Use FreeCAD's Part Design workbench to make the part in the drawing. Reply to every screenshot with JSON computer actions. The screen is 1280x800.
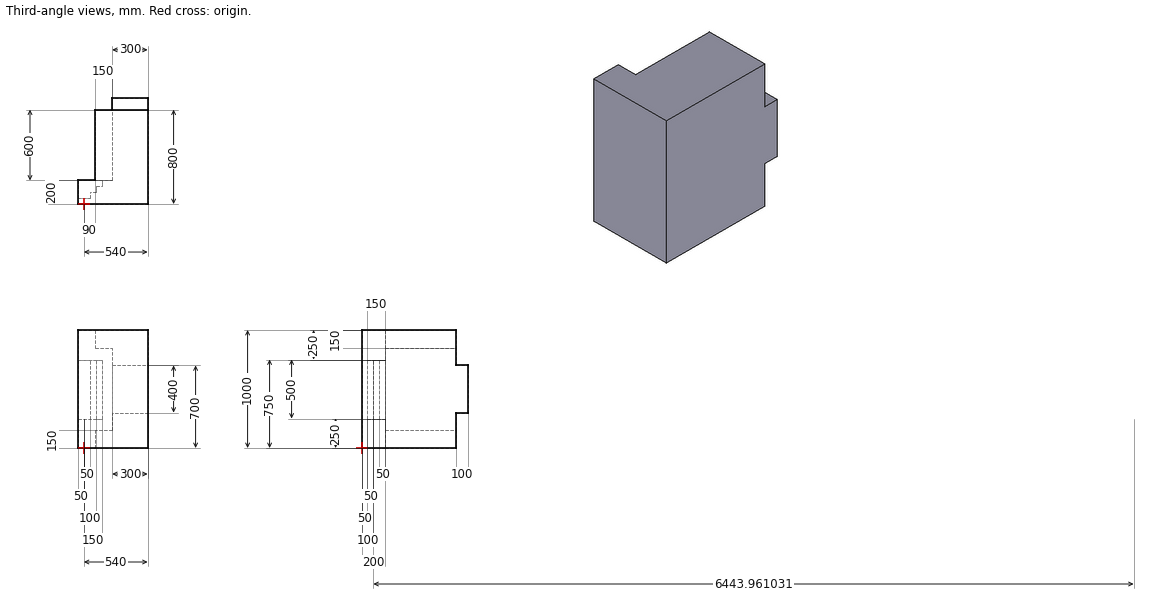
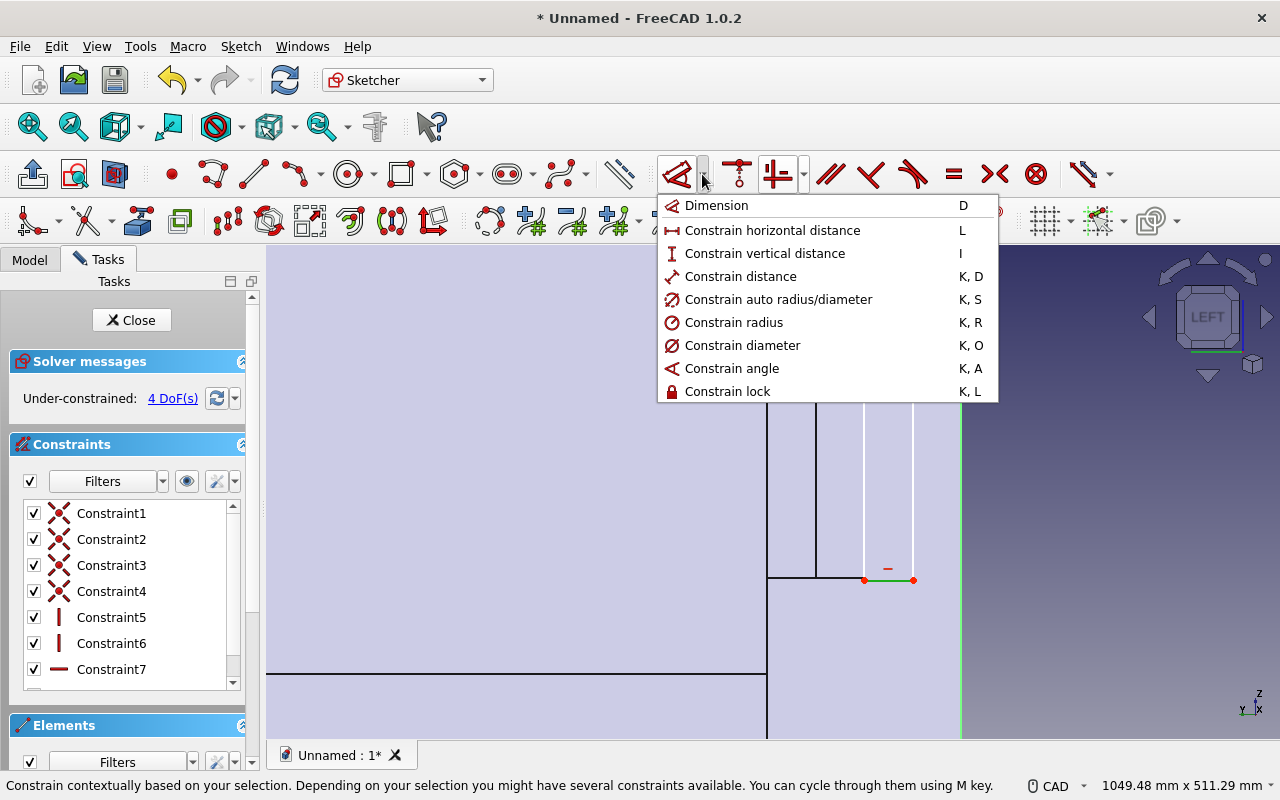
{"action": "left_click", "coordinate": [828, 230]}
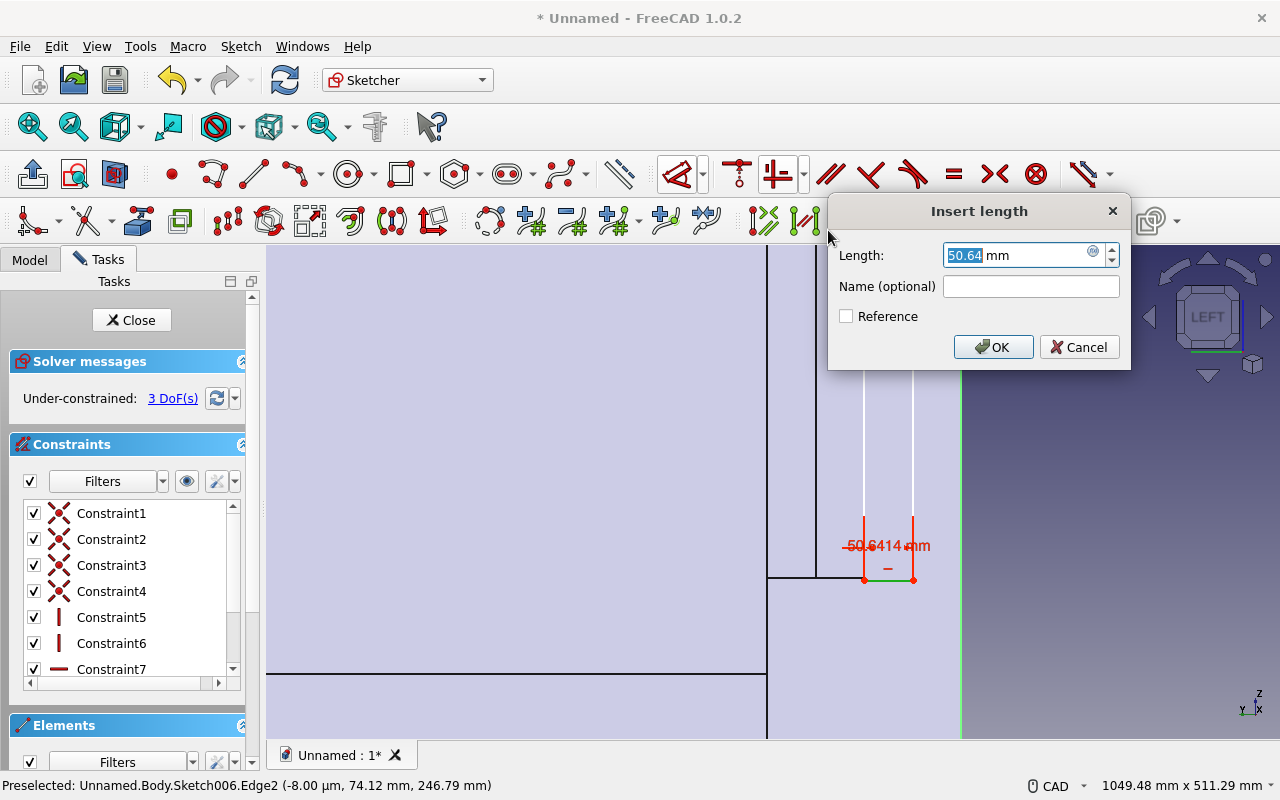
{"action": "type", "text": "50"}
{"action": "key", "text": "Return"}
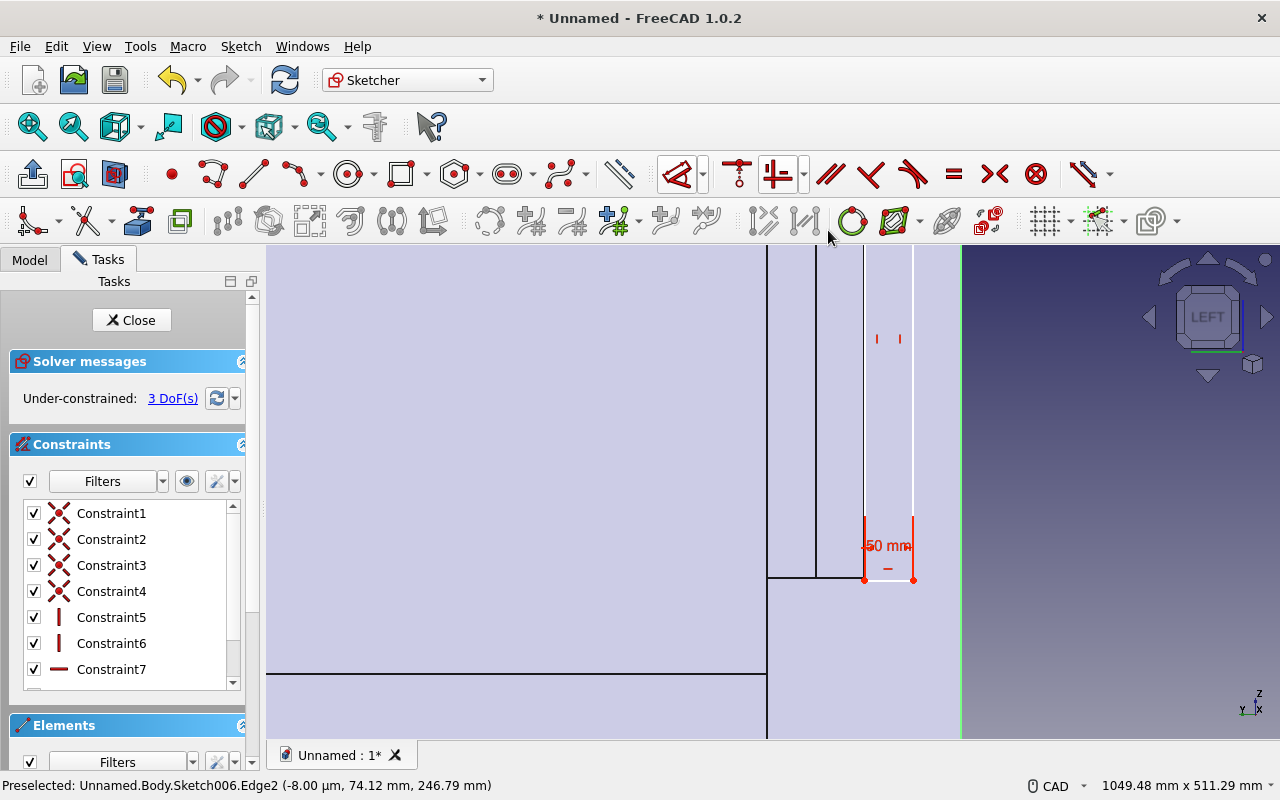
{"action": "left_click", "coordinate": [865, 436]}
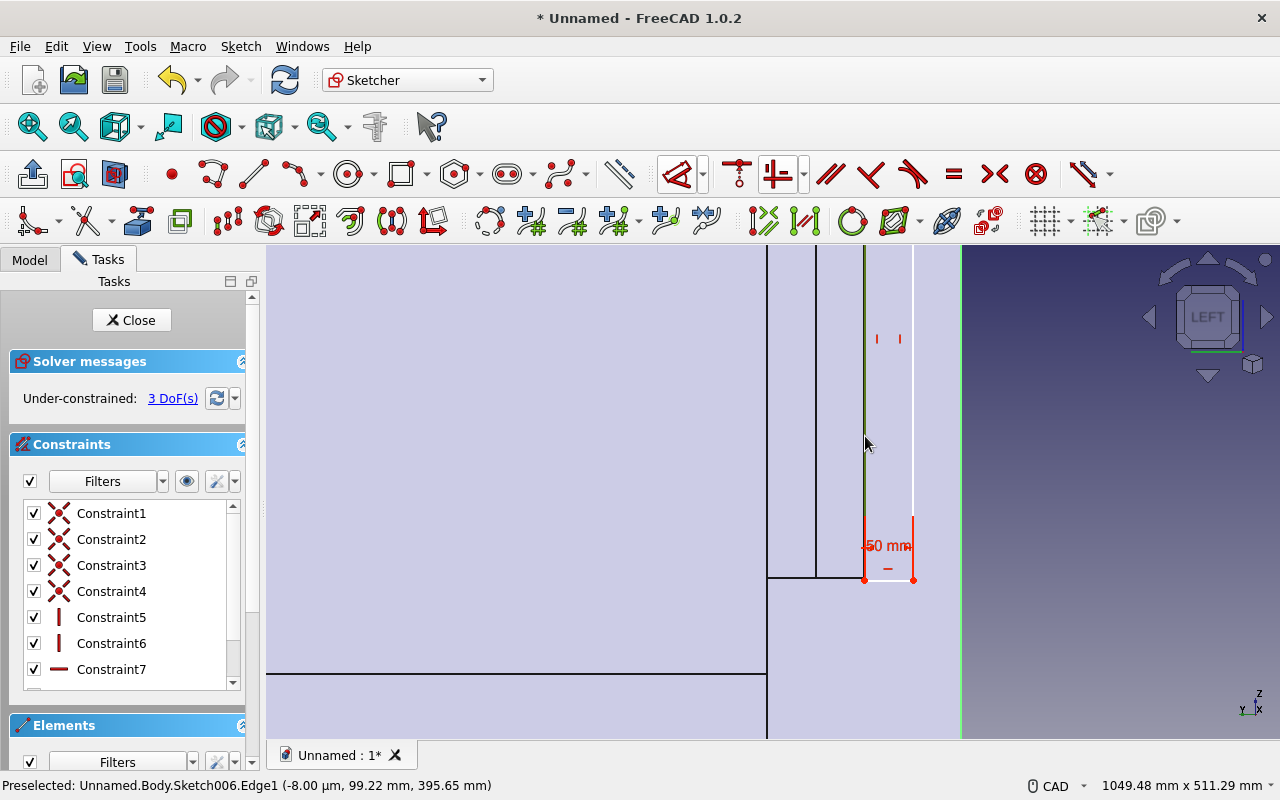
{"action": "key", "text": "i"}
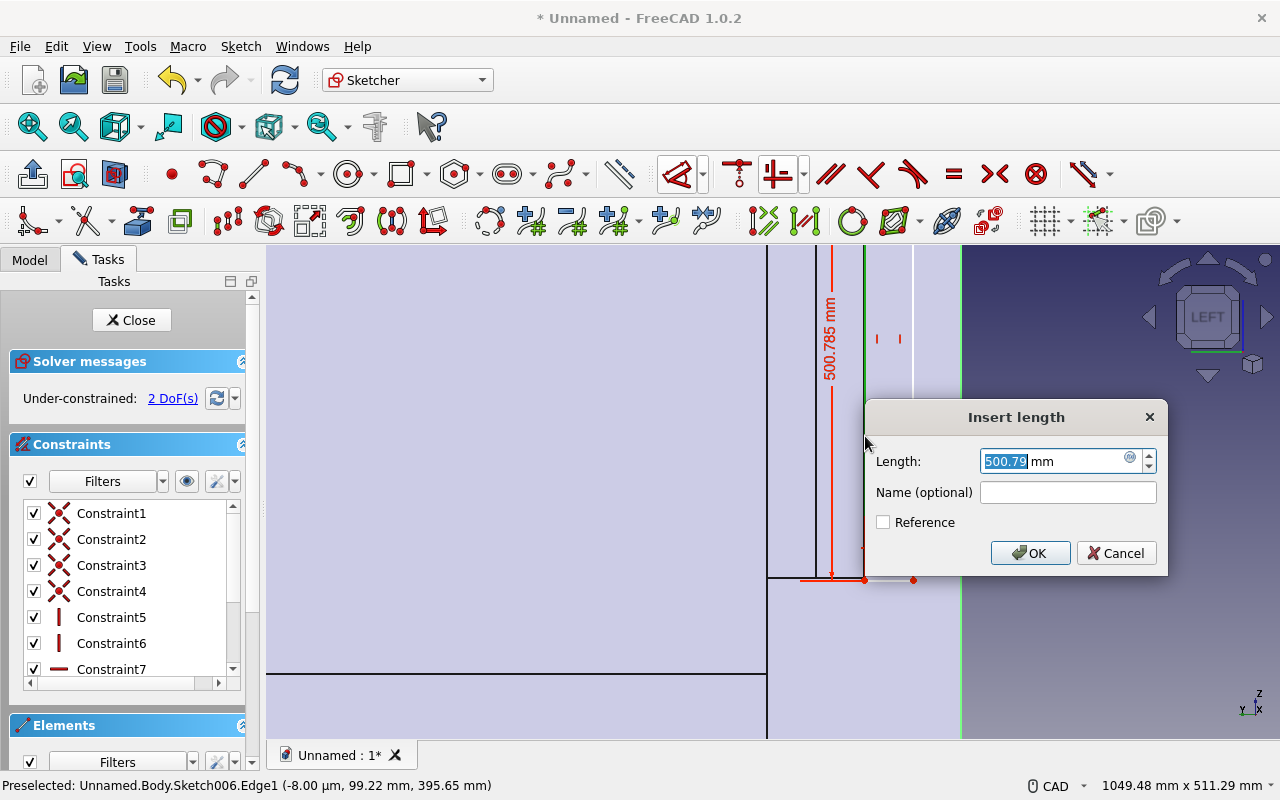
{"action": "type", "text": "500"}
{"action": "key", "text": "Return"}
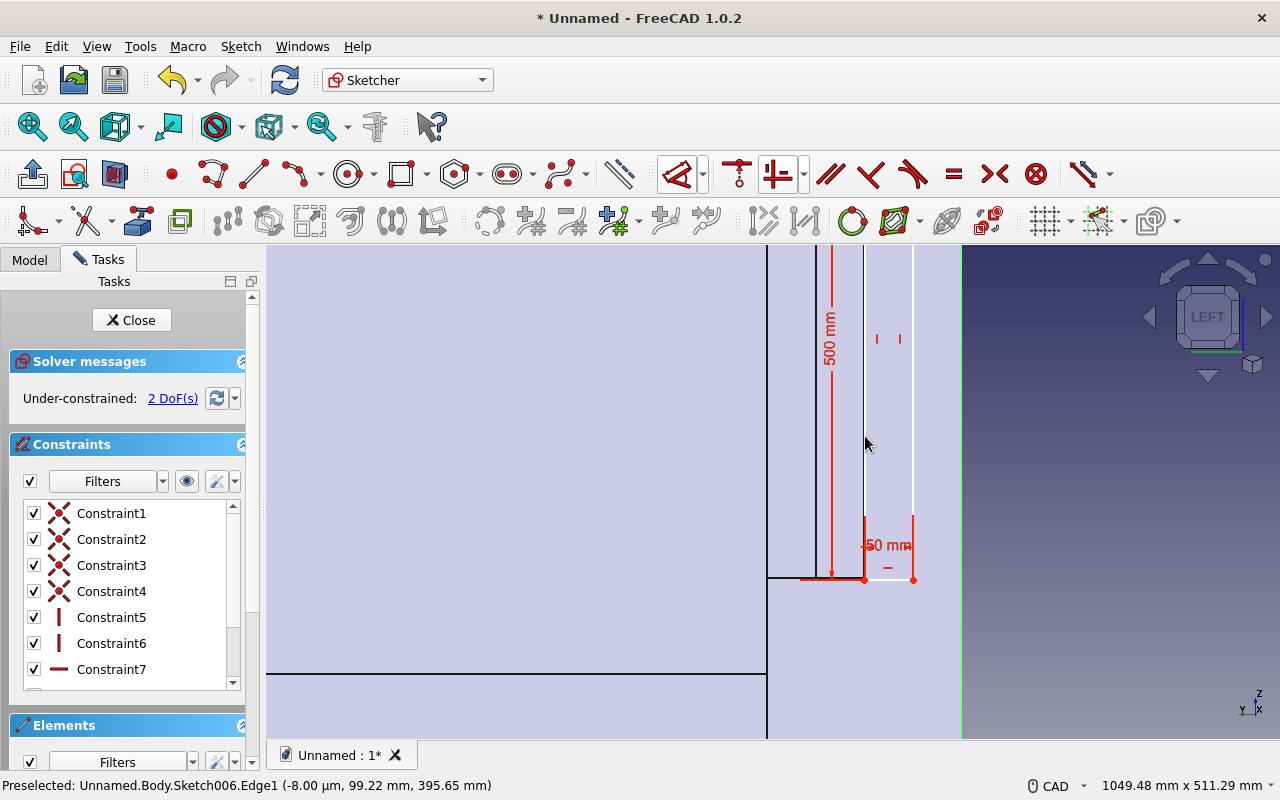
{"action": "left_click", "coordinate": [913, 580]}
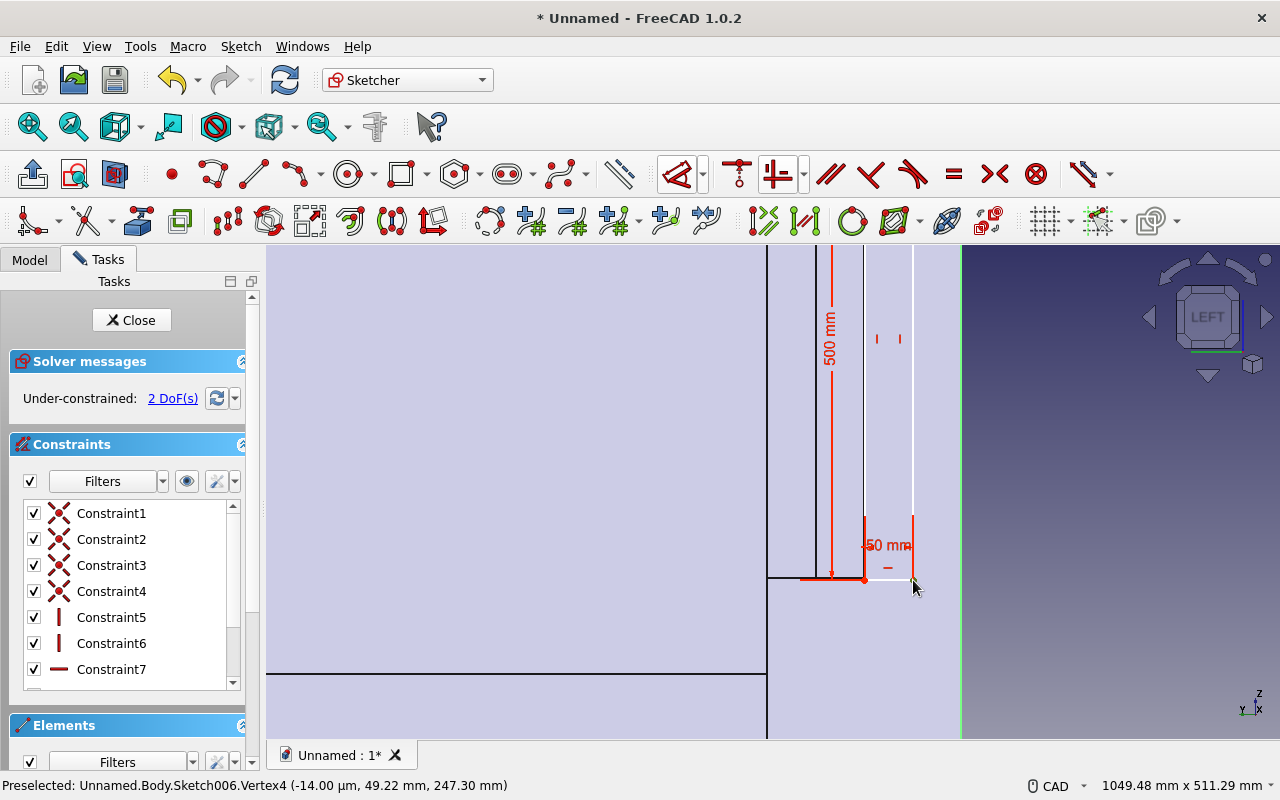
{"action": "left_click", "coordinate": [702, 174]}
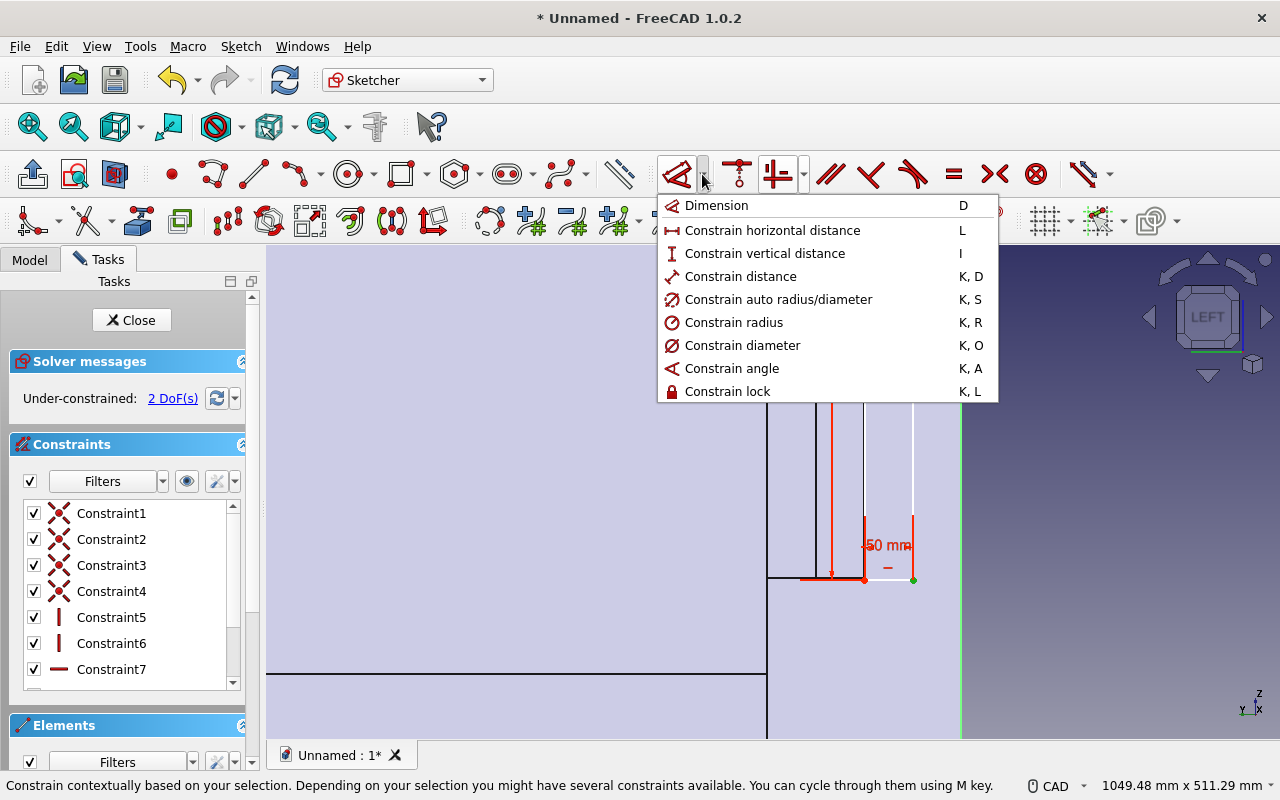
{"action": "left_click", "coordinate": [828, 230]}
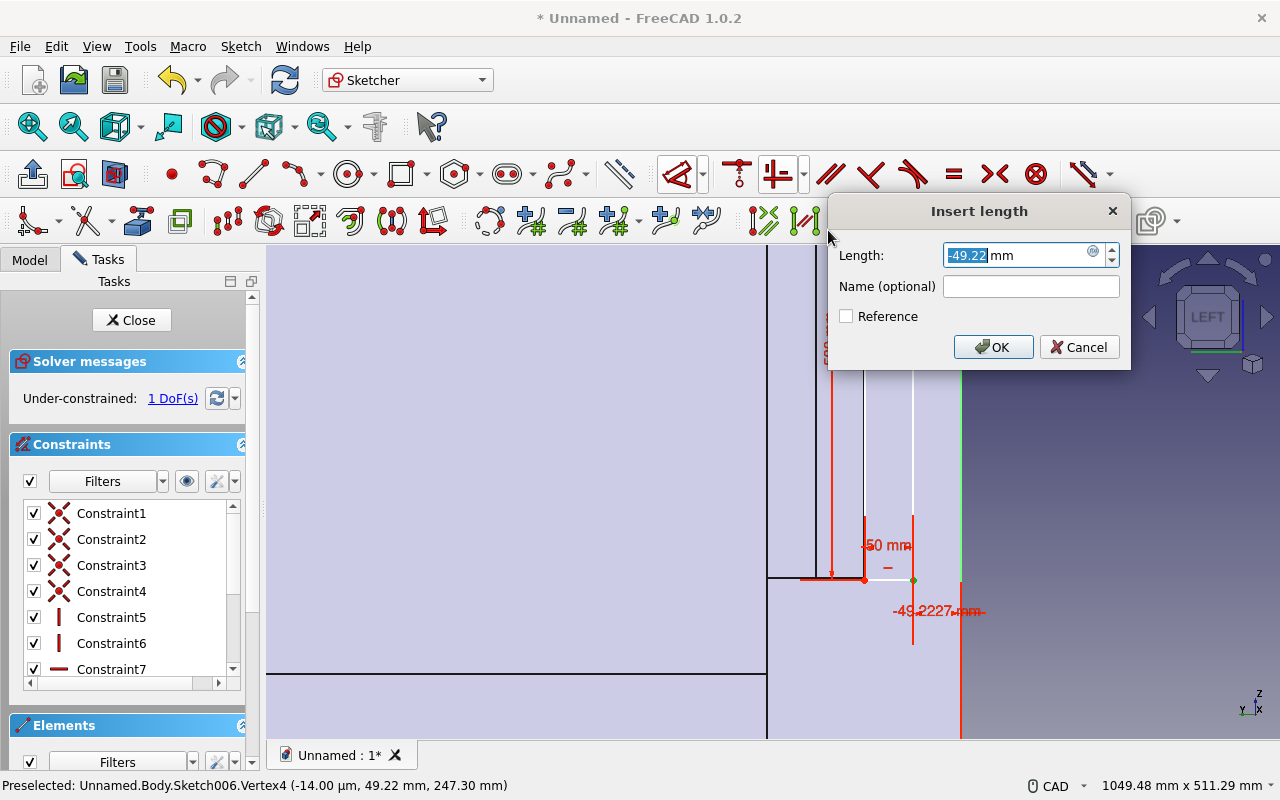
{"action": "type", "text": "-50"}
{"action": "key", "text": "Return"}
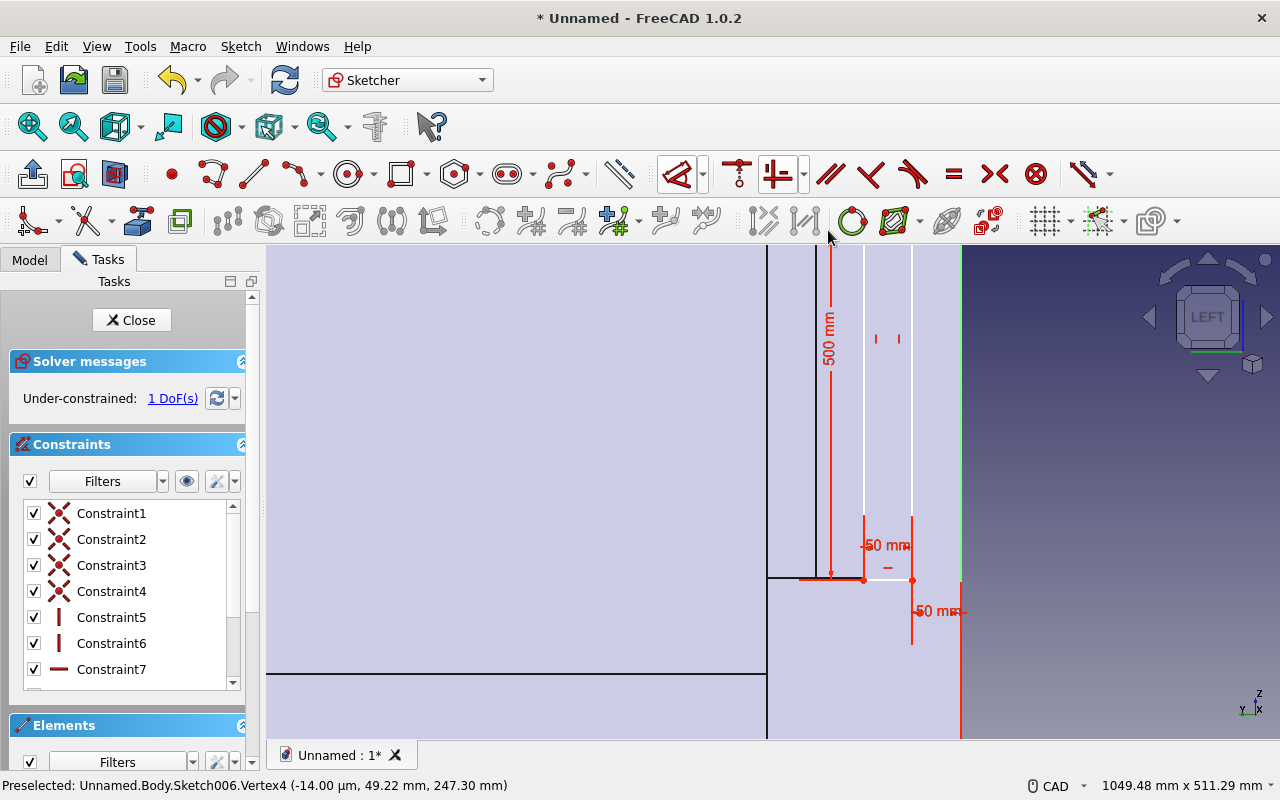
{"action": "scroll", "coordinate": [535, 521], "scroll_direction": "down", "scroll_amount": 4}